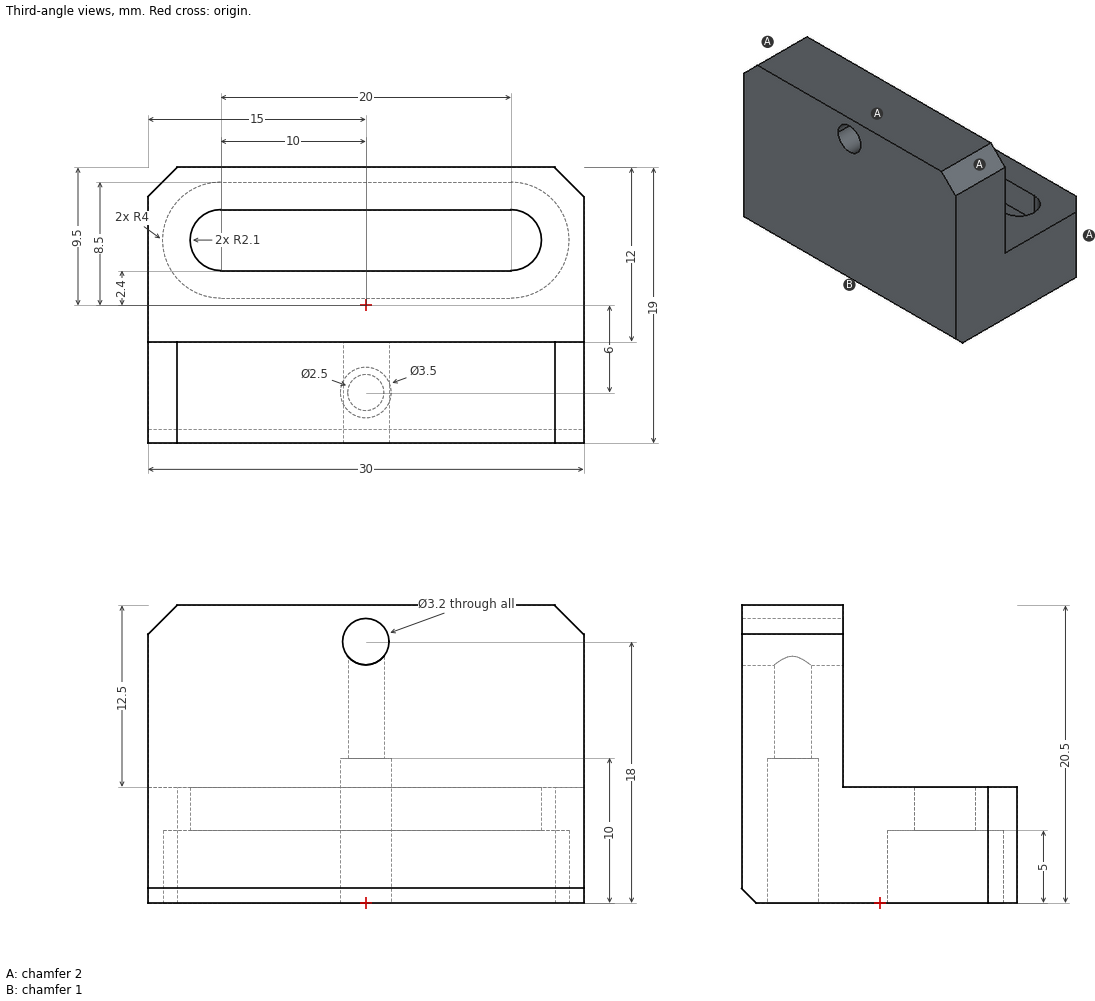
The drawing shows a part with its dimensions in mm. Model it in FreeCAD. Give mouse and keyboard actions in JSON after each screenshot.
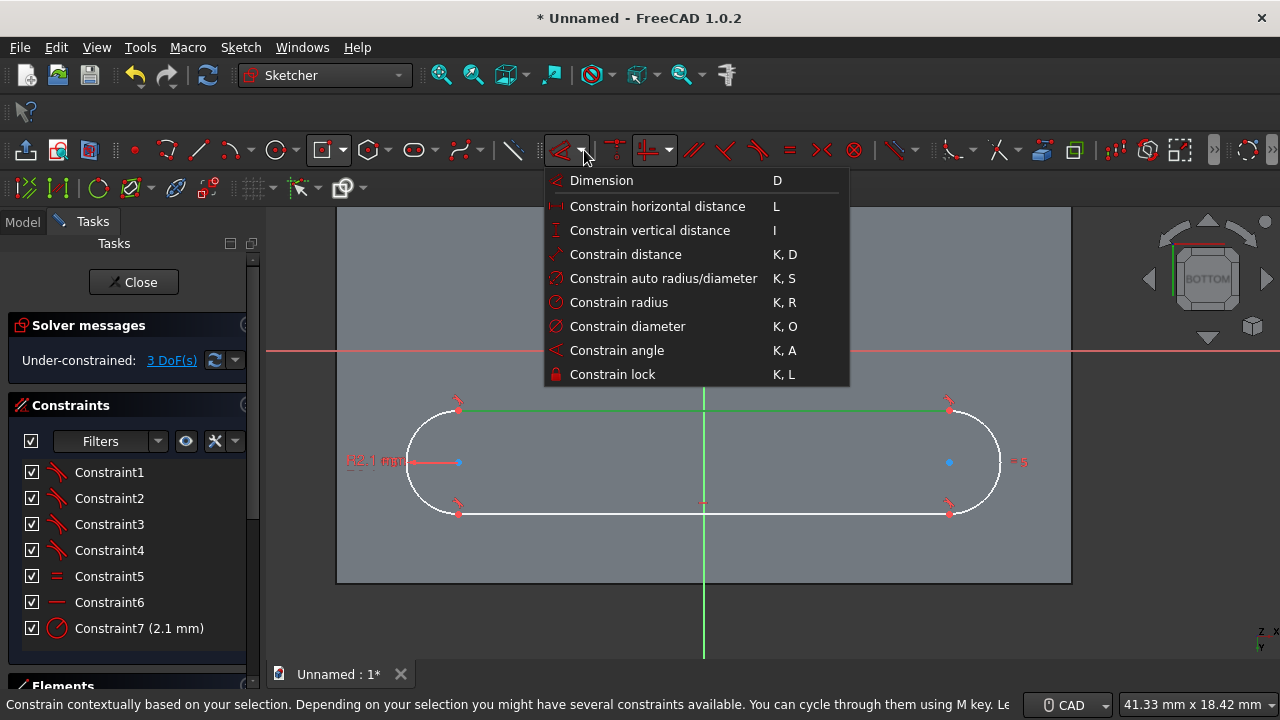
{"action": "left_click", "coordinate": [697, 206]}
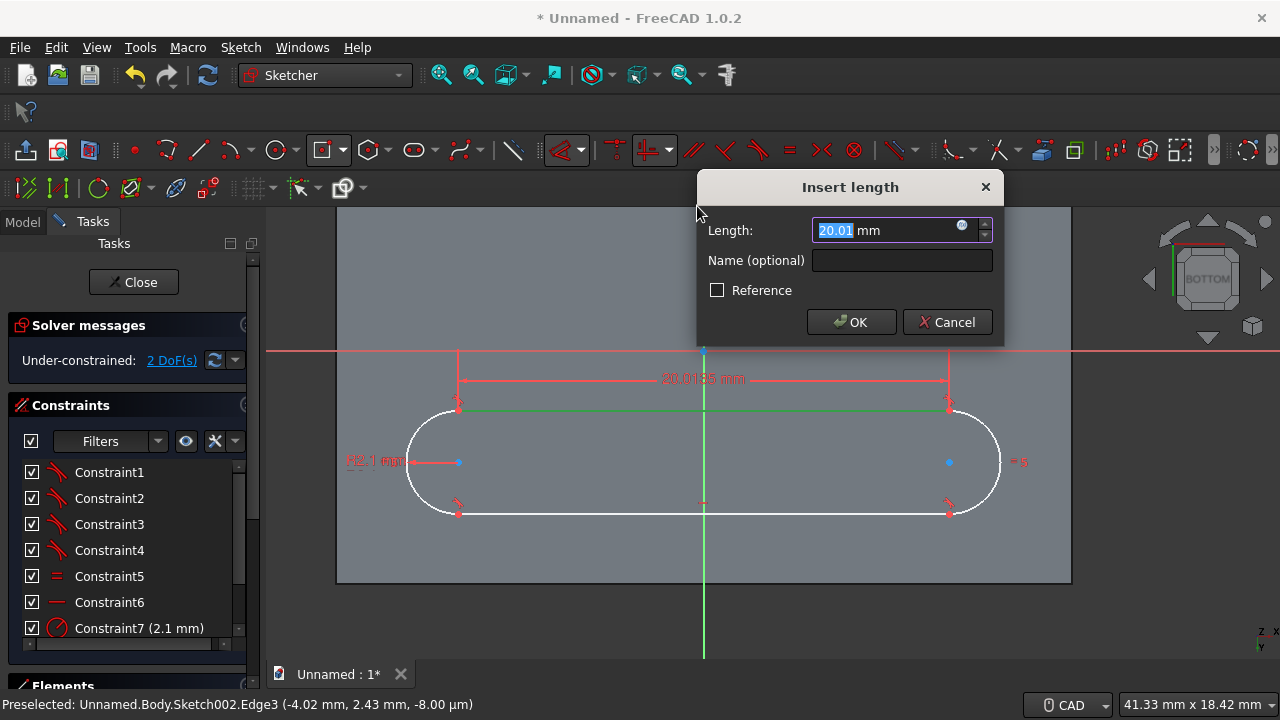
{"action": "type", "text": "20"}
{"action": "key", "text": "Return"}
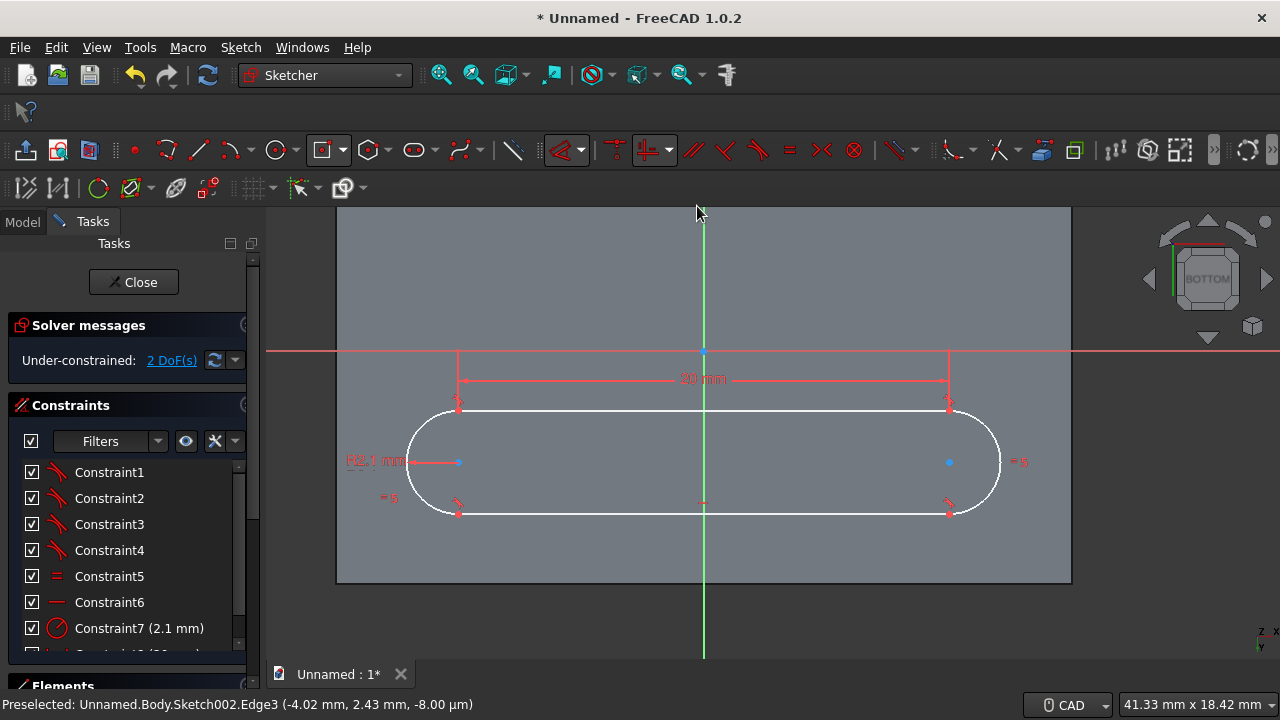
{"action": "left_click", "coordinate": [458, 411]}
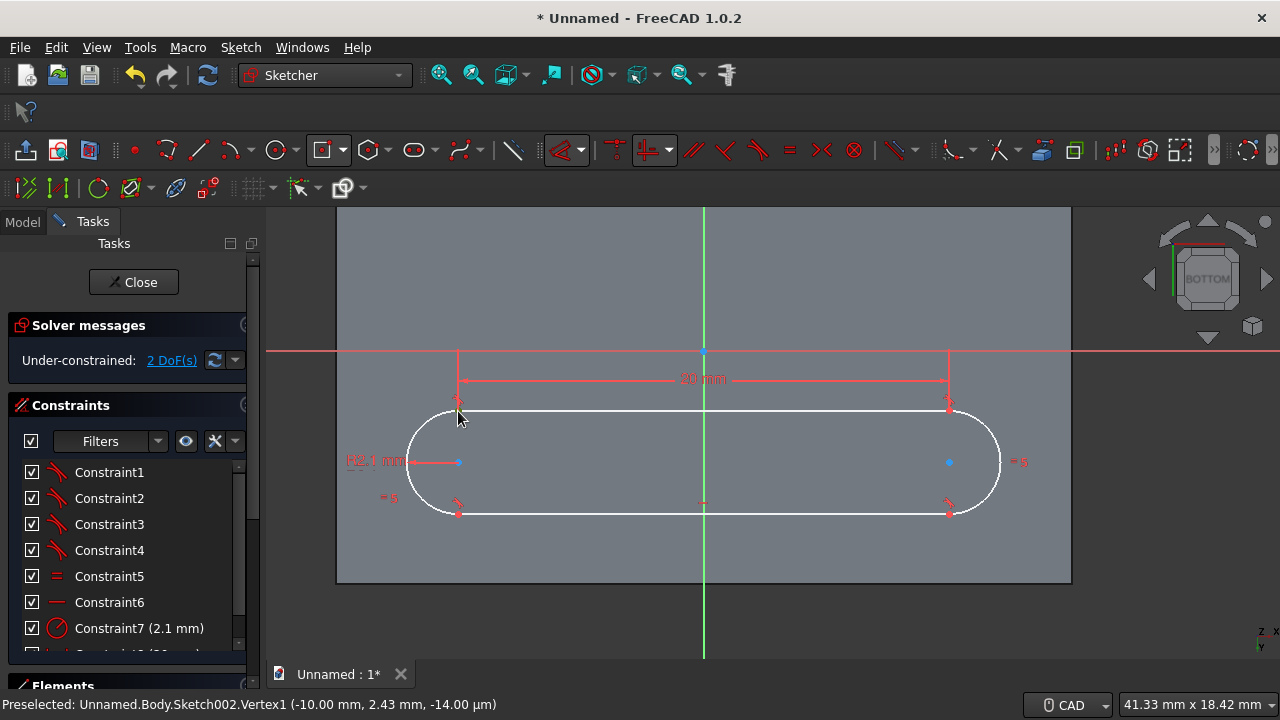
{"action": "key", "text": "l"}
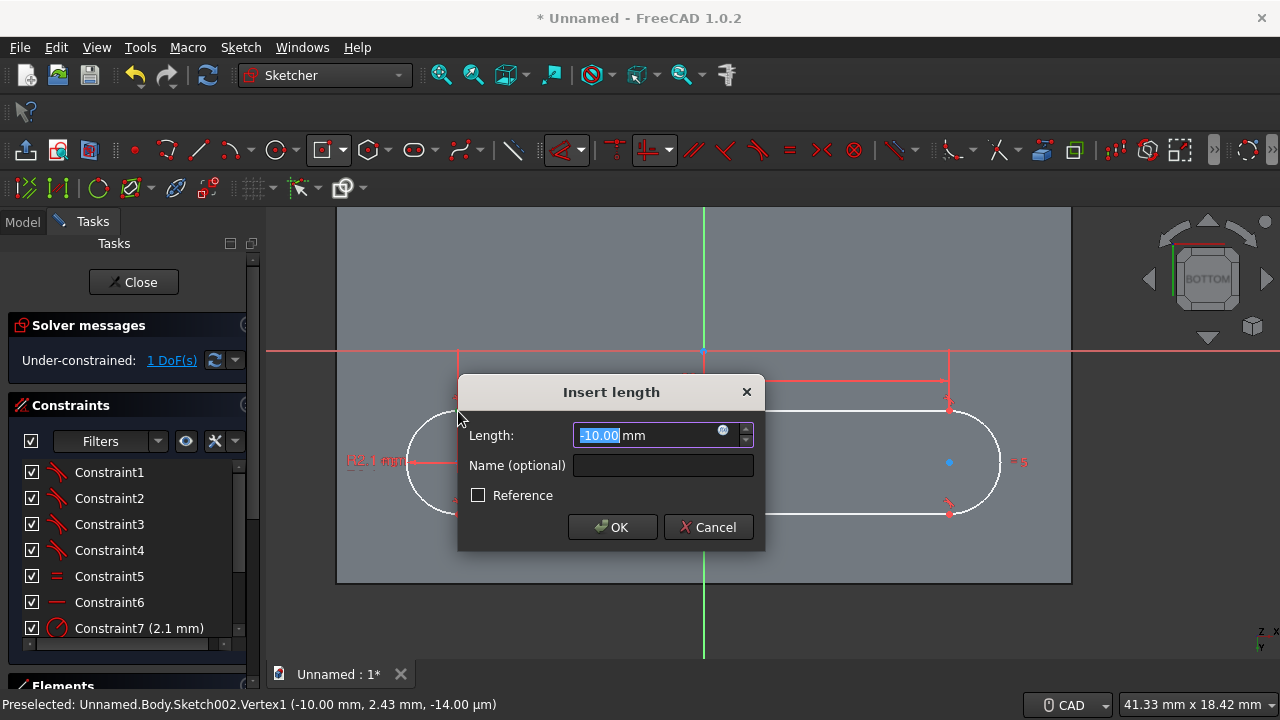
{"action": "type", "text": "-10"}
{"action": "key", "text": "Return"}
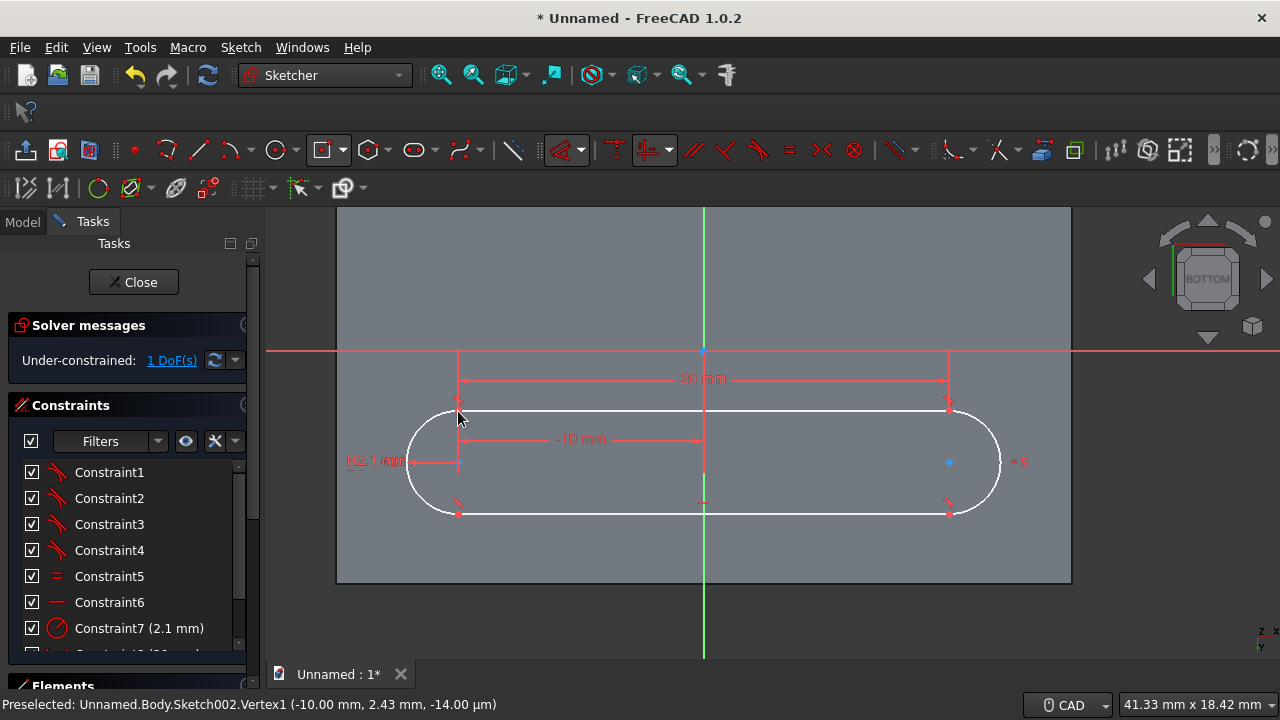
{"action": "left_click", "coordinate": [458, 411]}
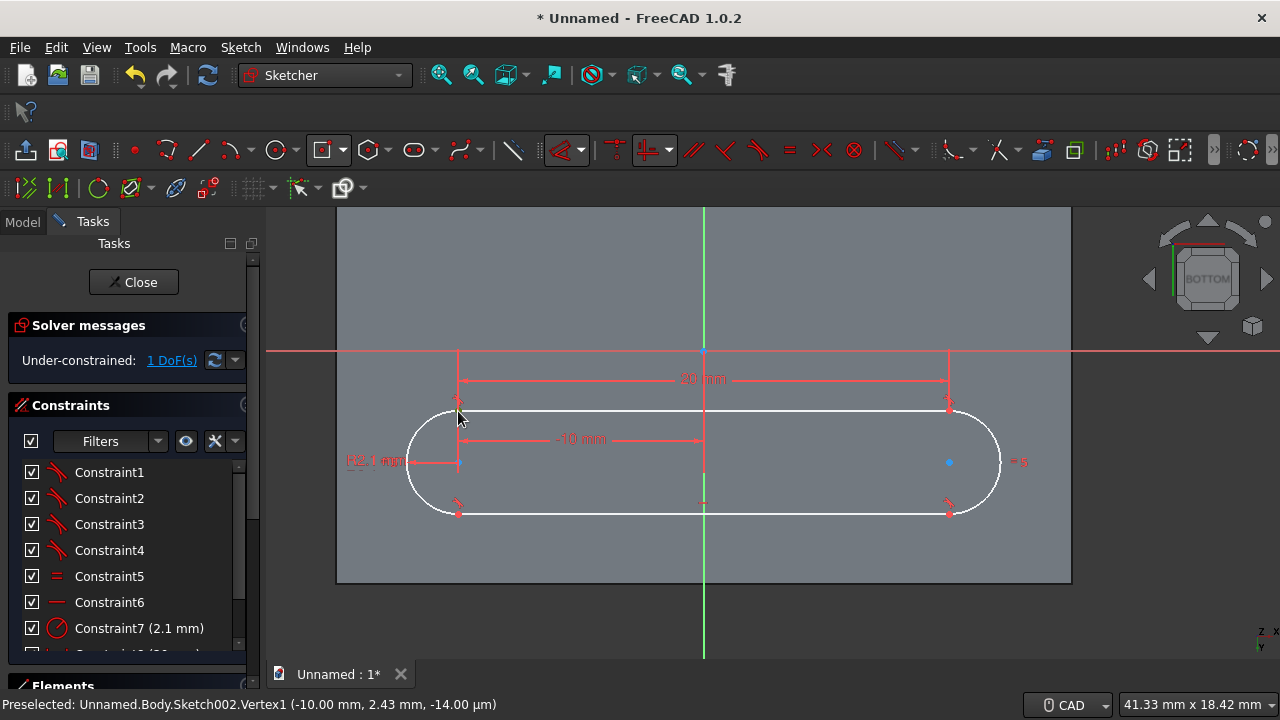
{"action": "key", "text": "i"}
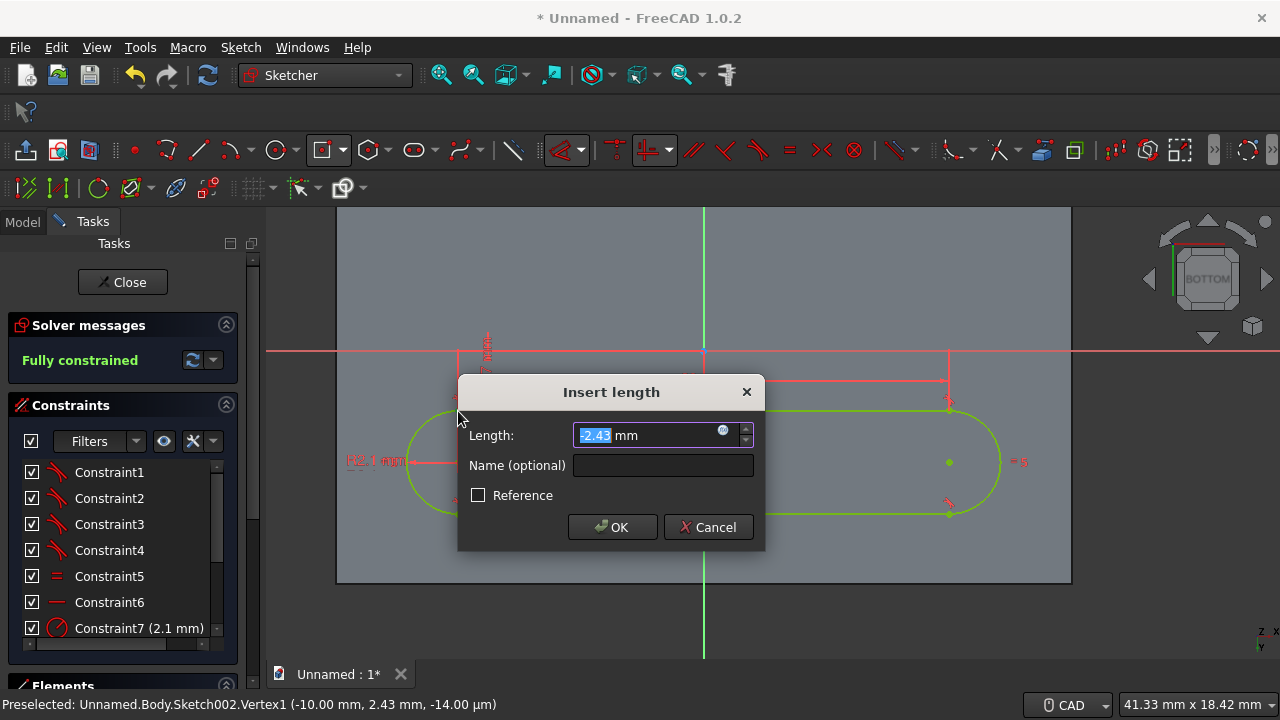
{"action": "type", "text": "-2.4"}
{"action": "key", "text": "Return"}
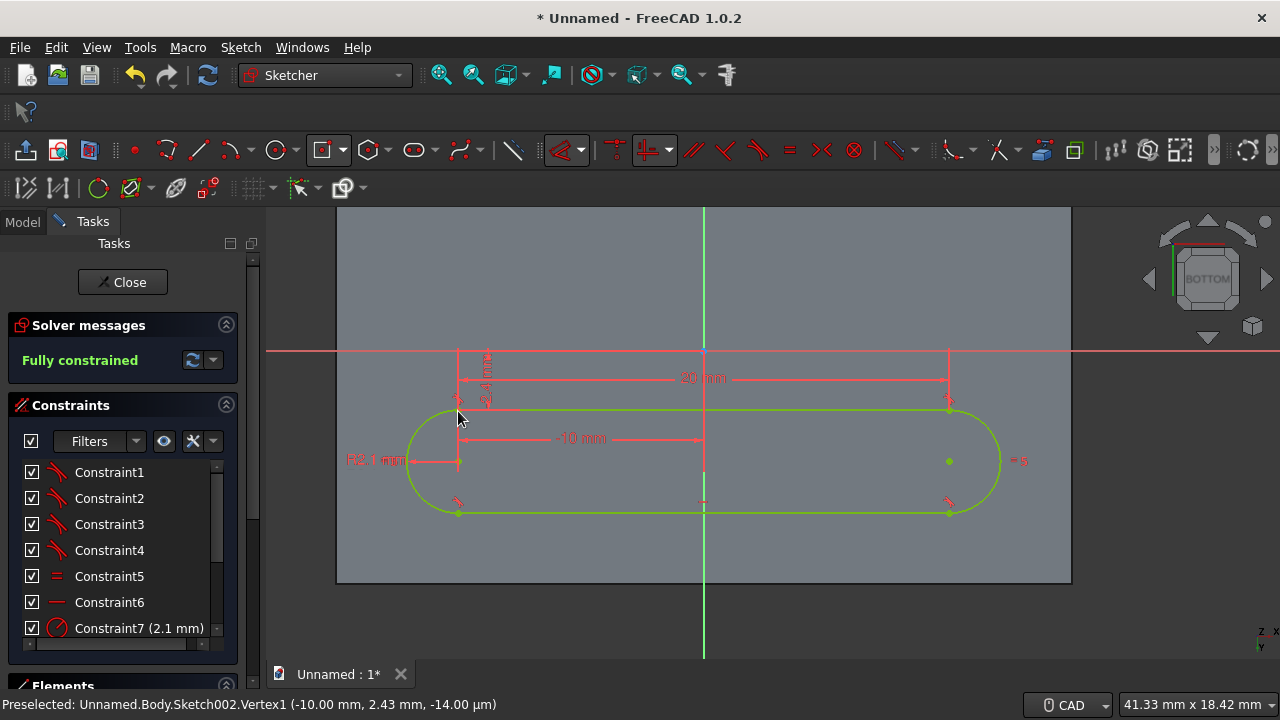
{"action": "left_click", "coordinate": [123, 282]}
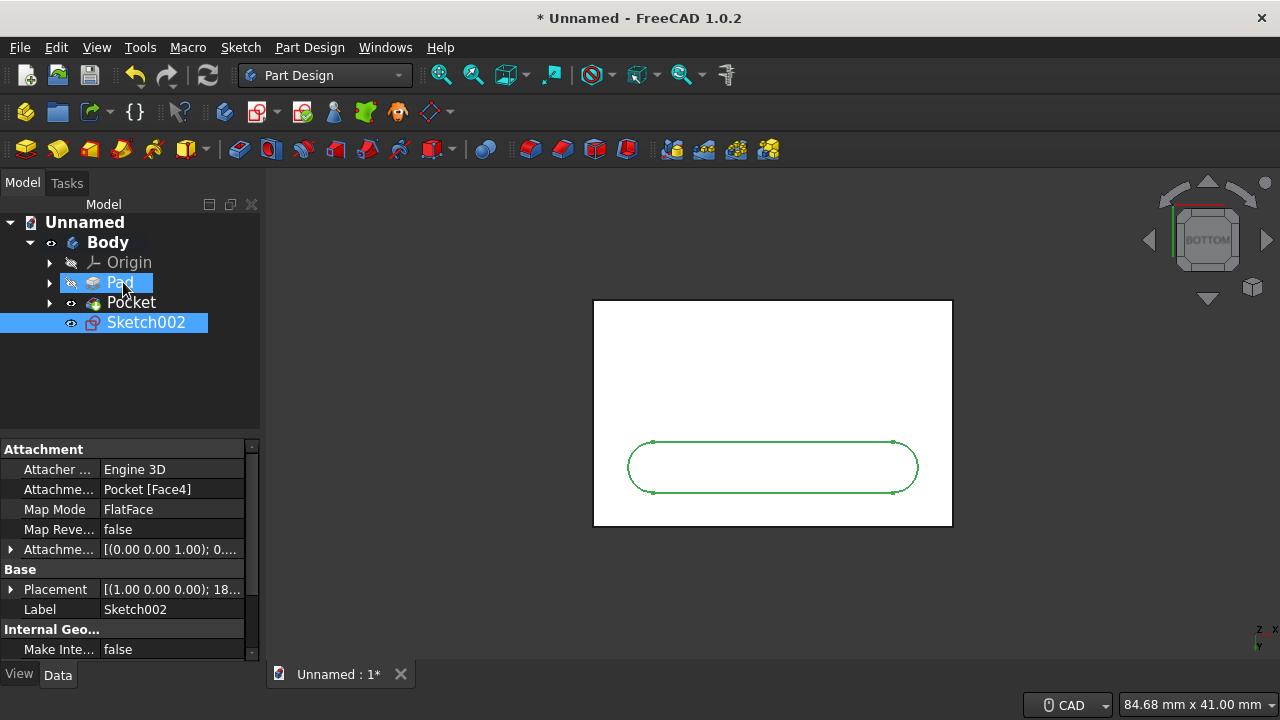
{"action": "left_click", "coordinate": [240, 150]}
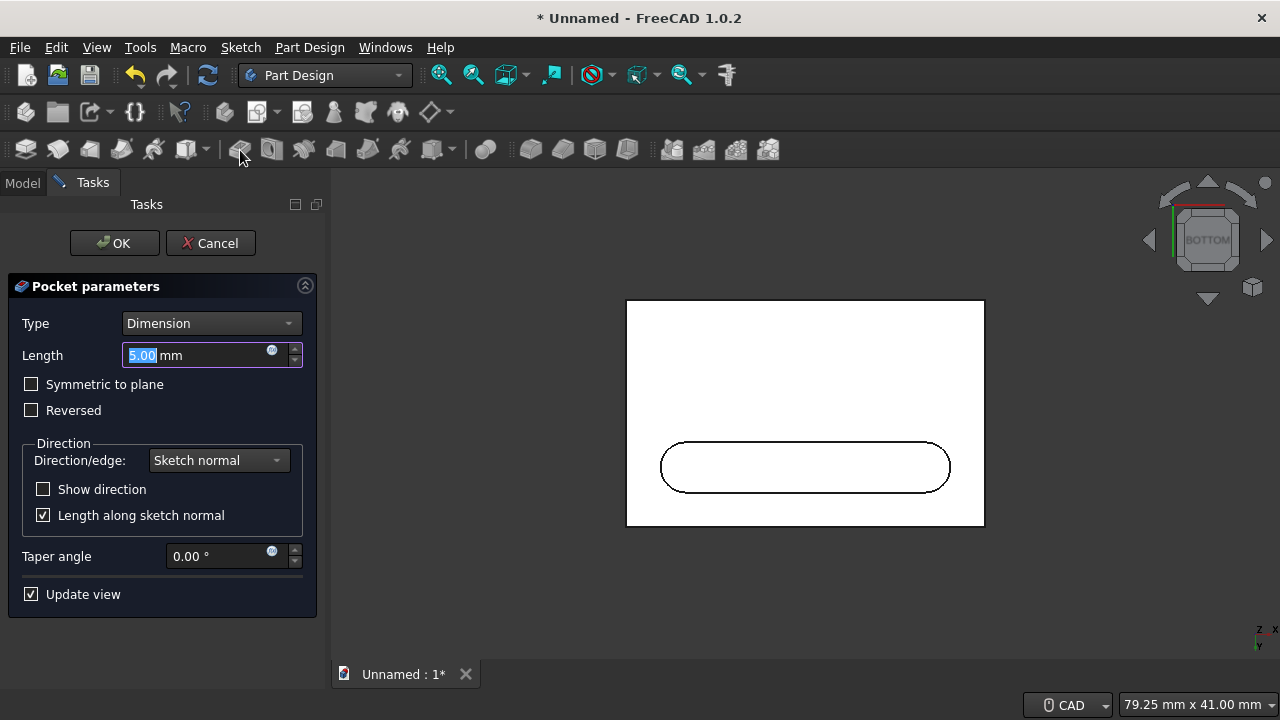
{"action": "left_click", "coordinate": [212, 324]}